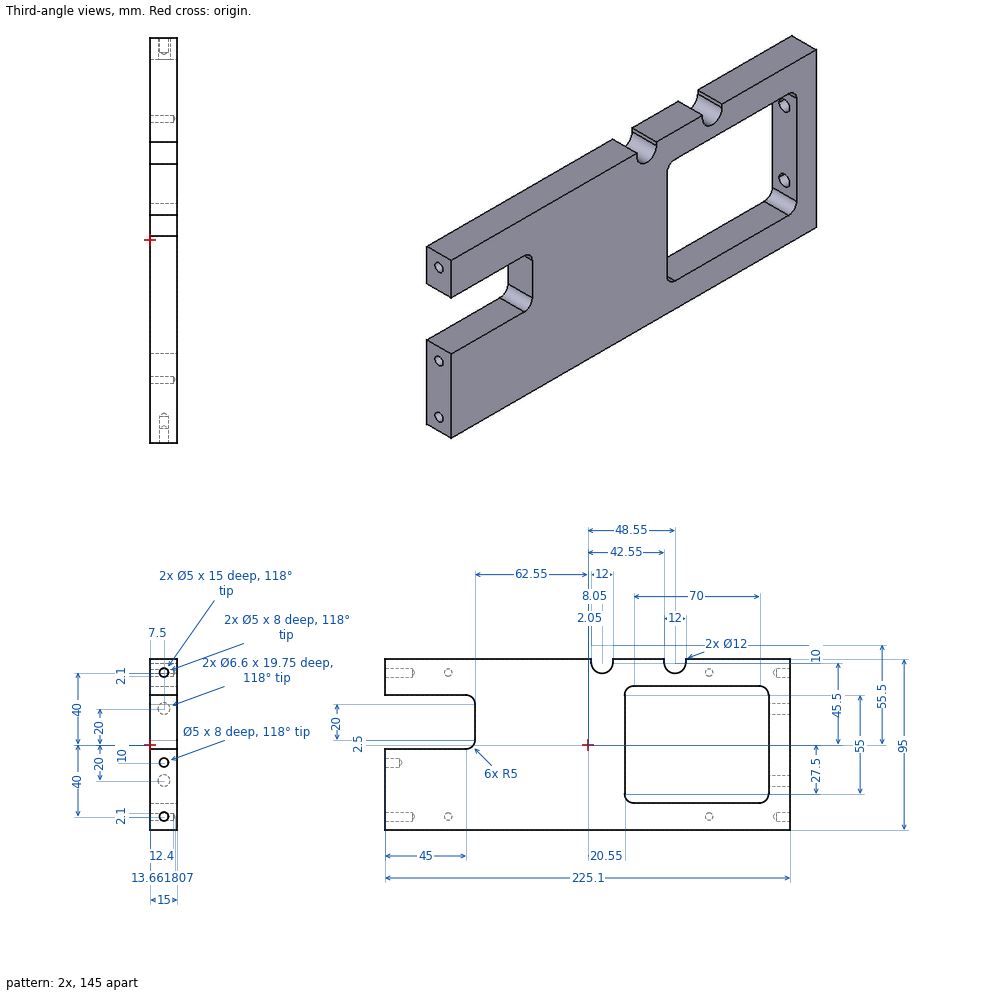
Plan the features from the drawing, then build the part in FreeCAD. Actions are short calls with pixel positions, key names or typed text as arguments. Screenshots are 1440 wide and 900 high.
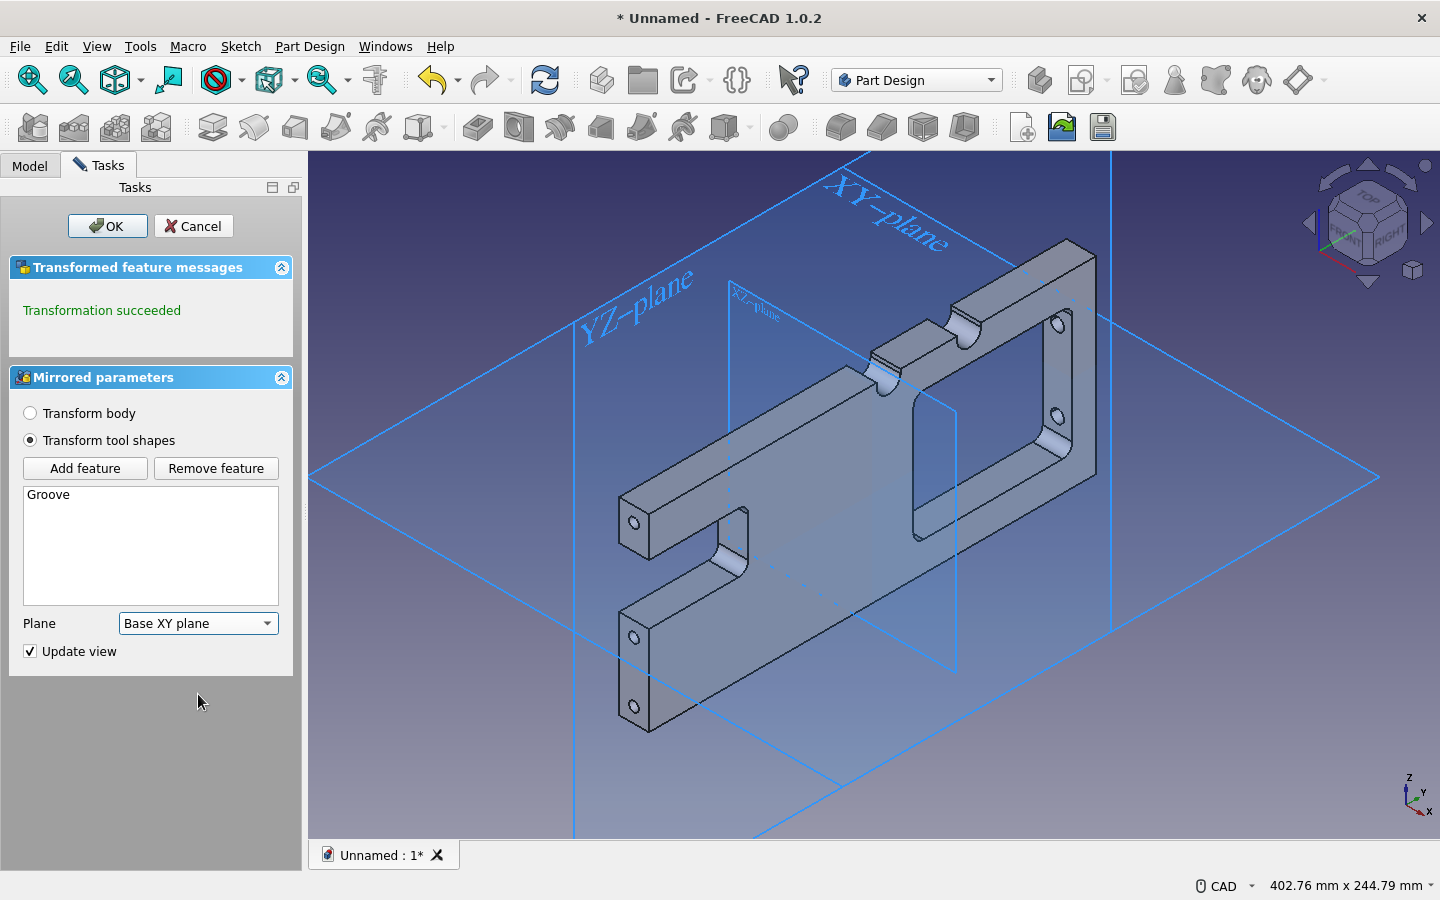
click(108, 226)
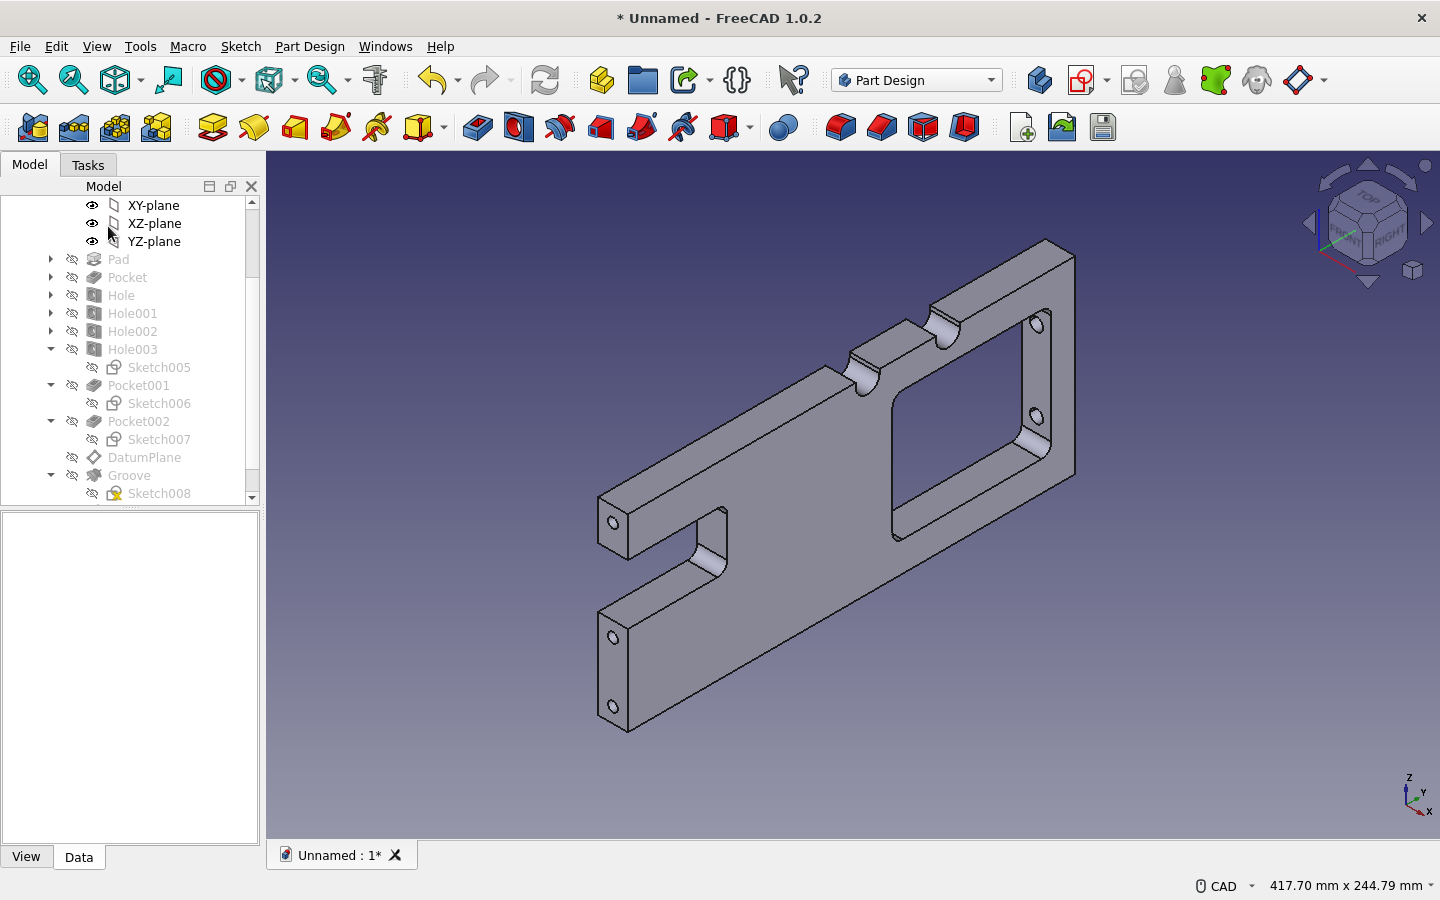
scroll(161, 345, down, 3)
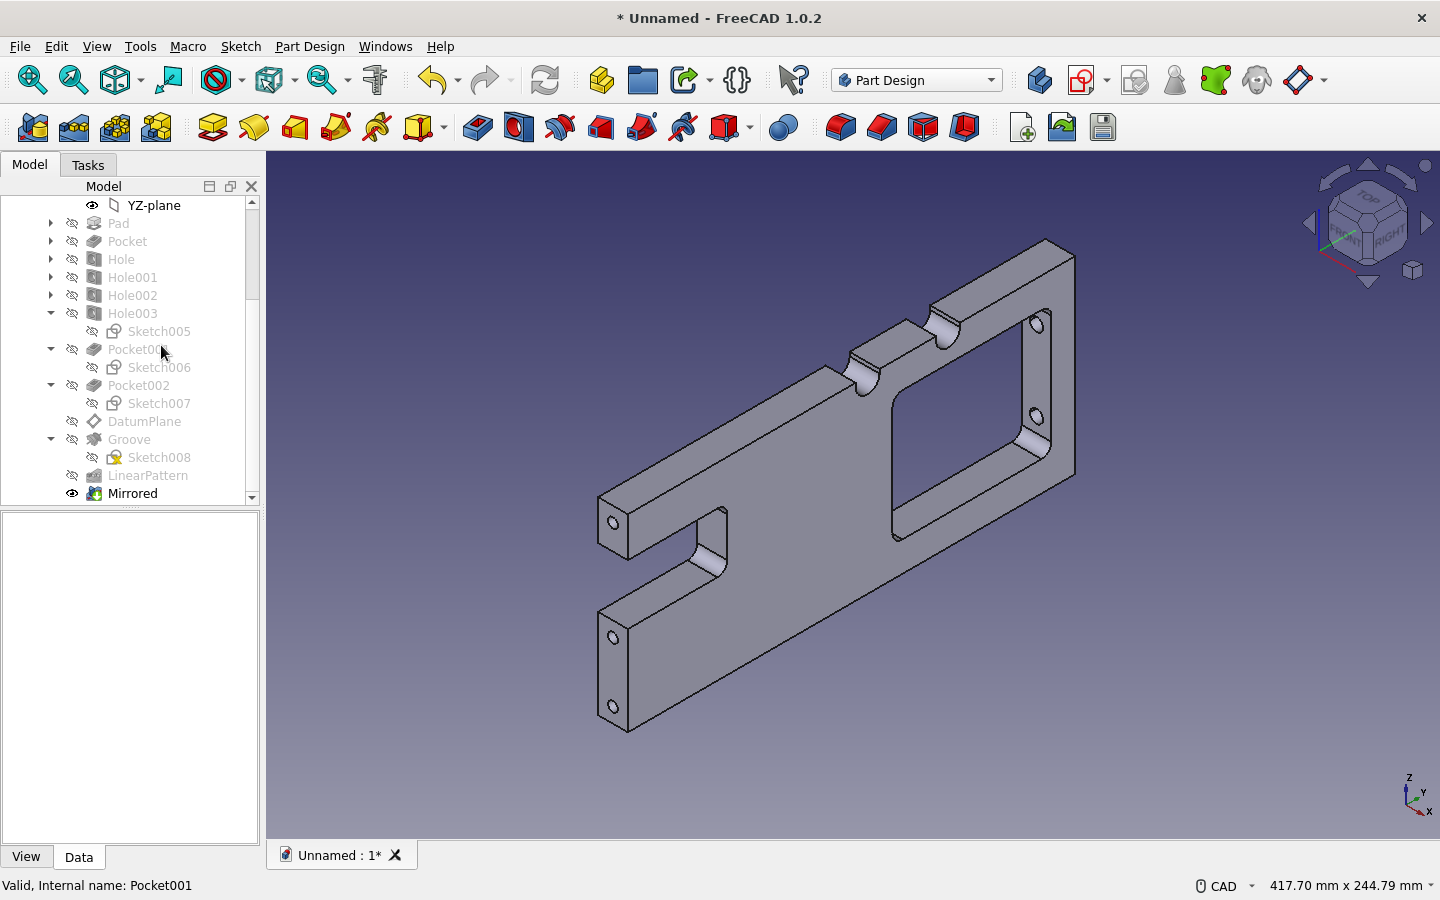
scroll(161, 345, up, 15)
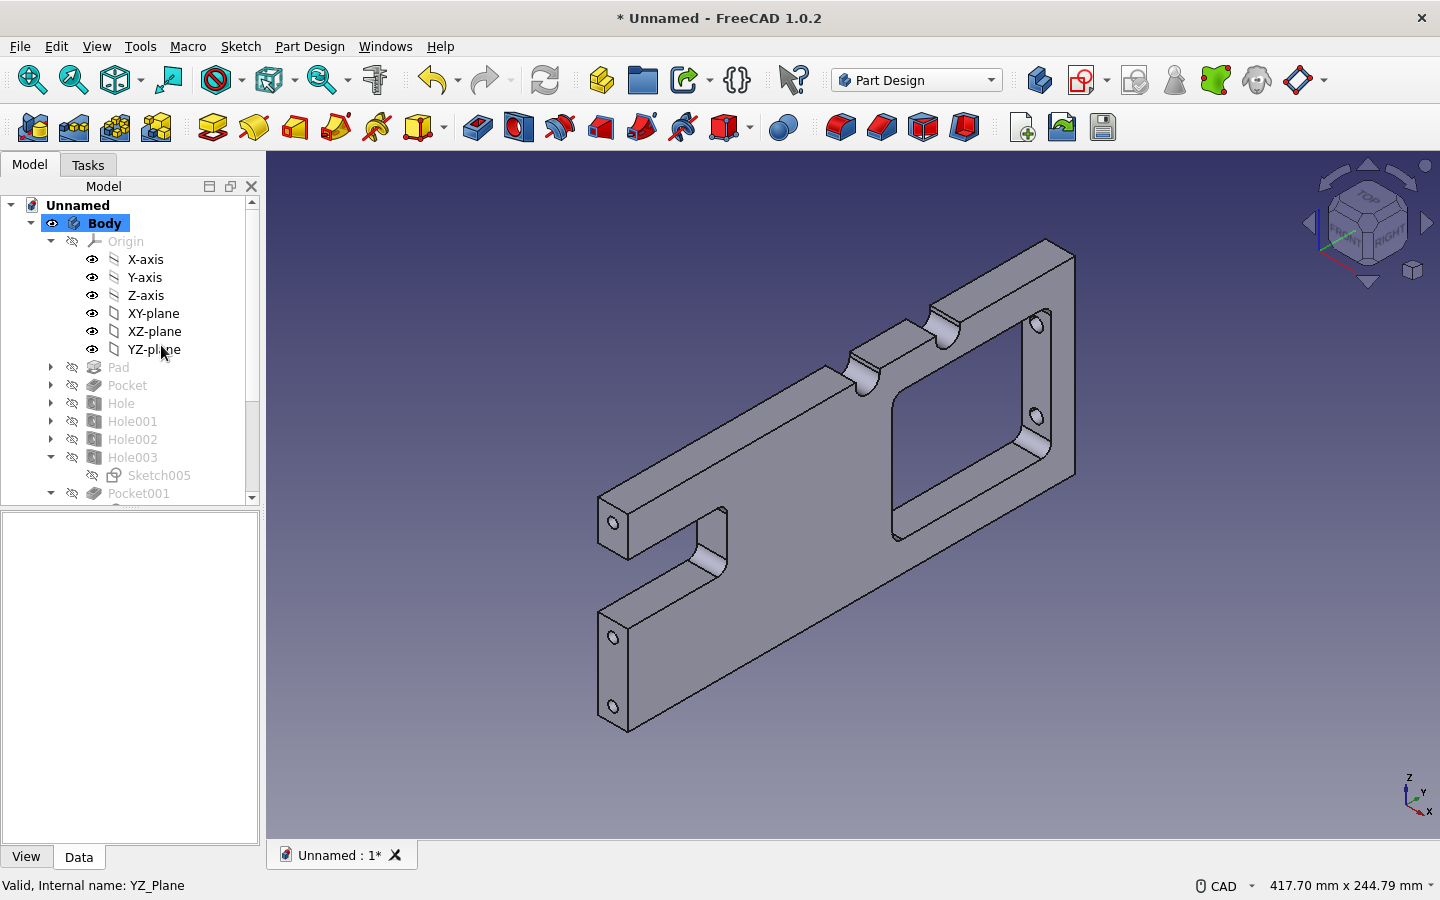
click(137, 331)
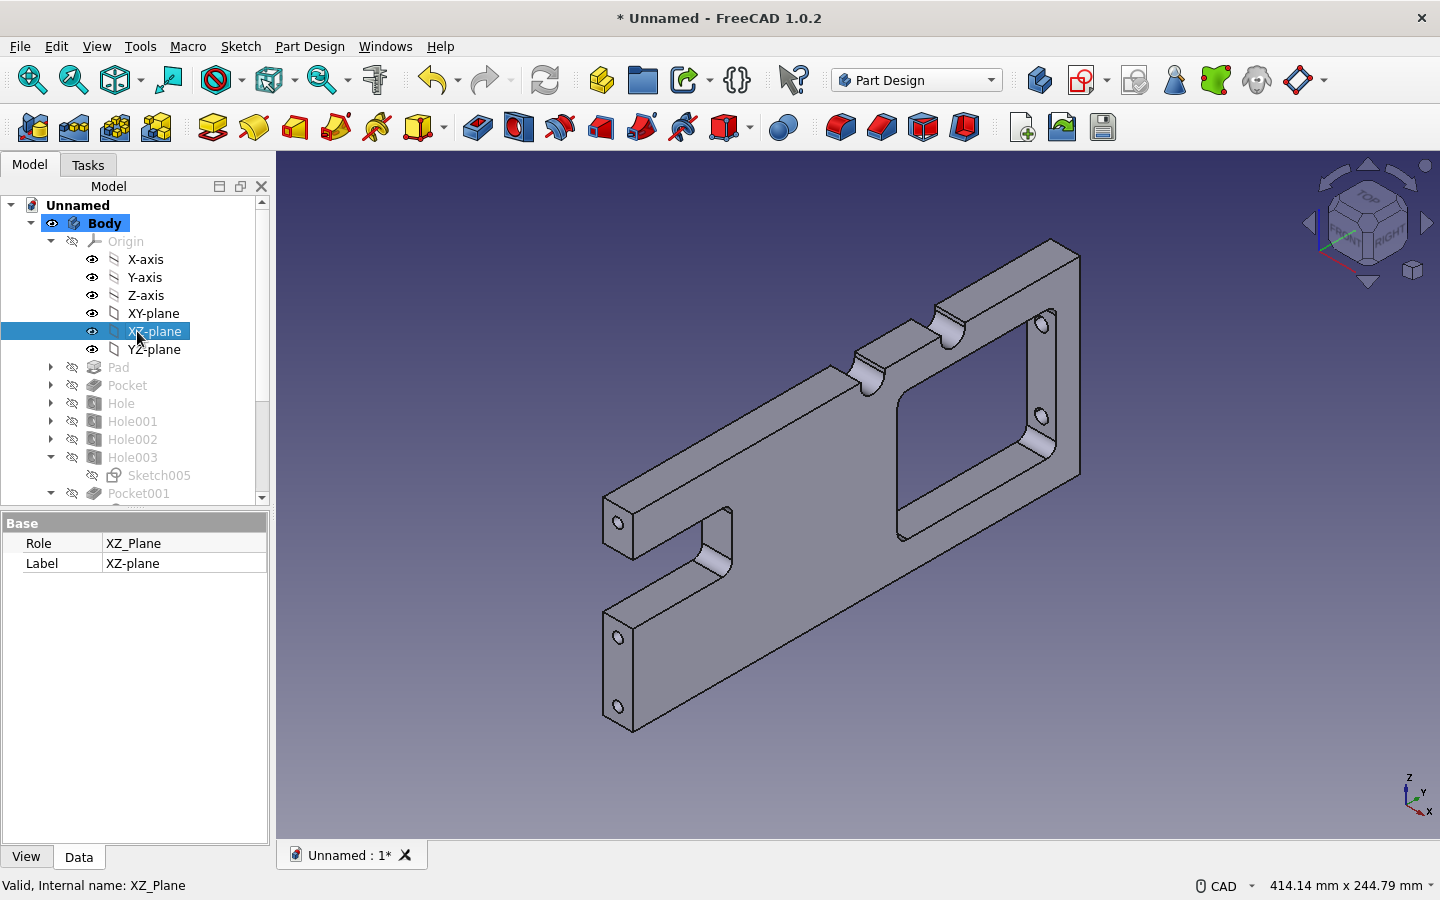
click(1298, 80)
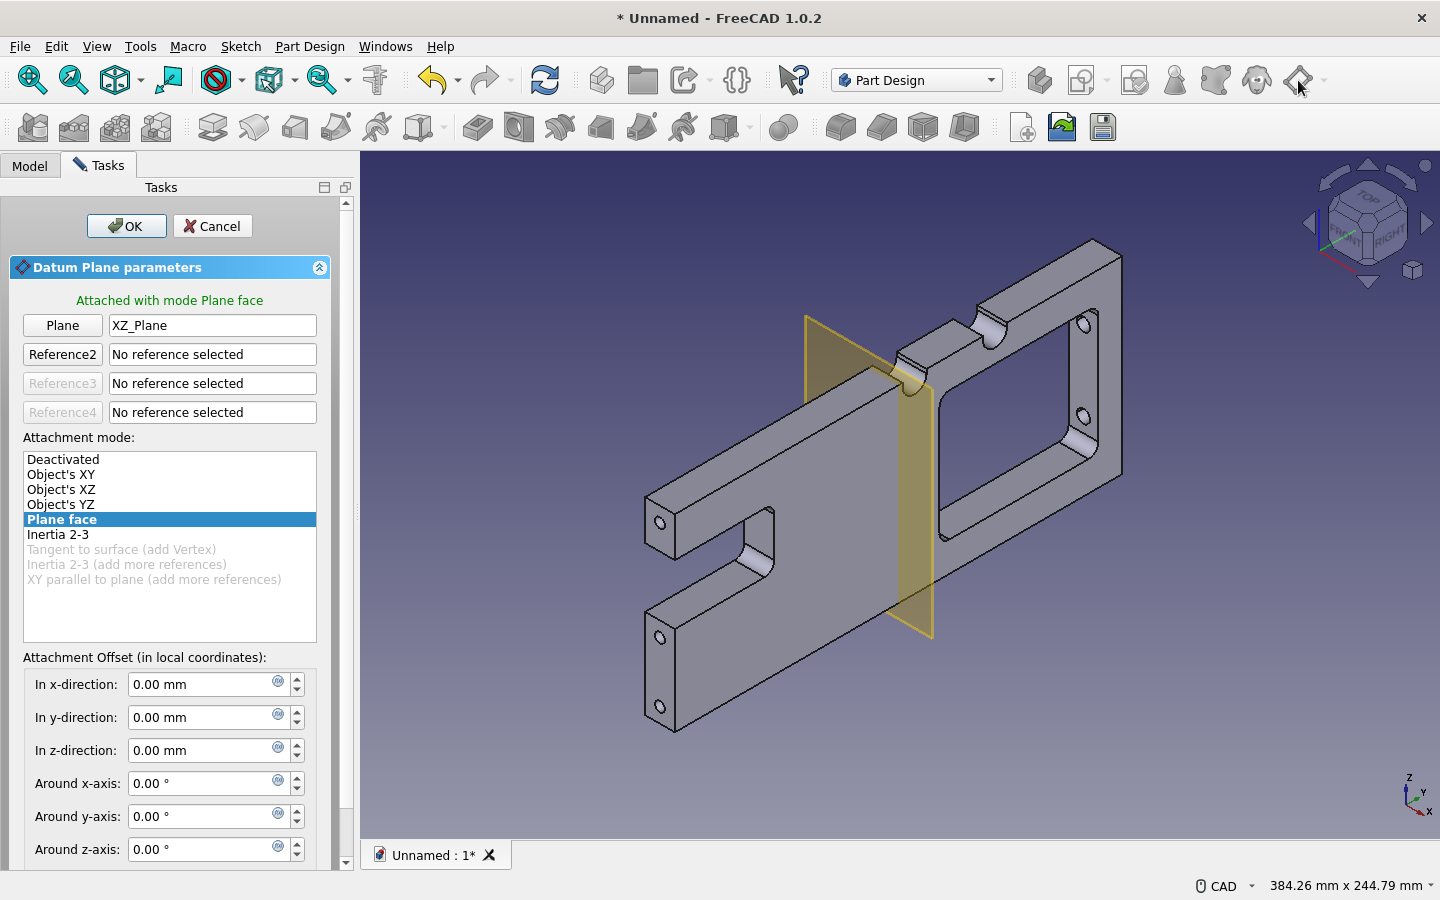
triple_click(210, 750)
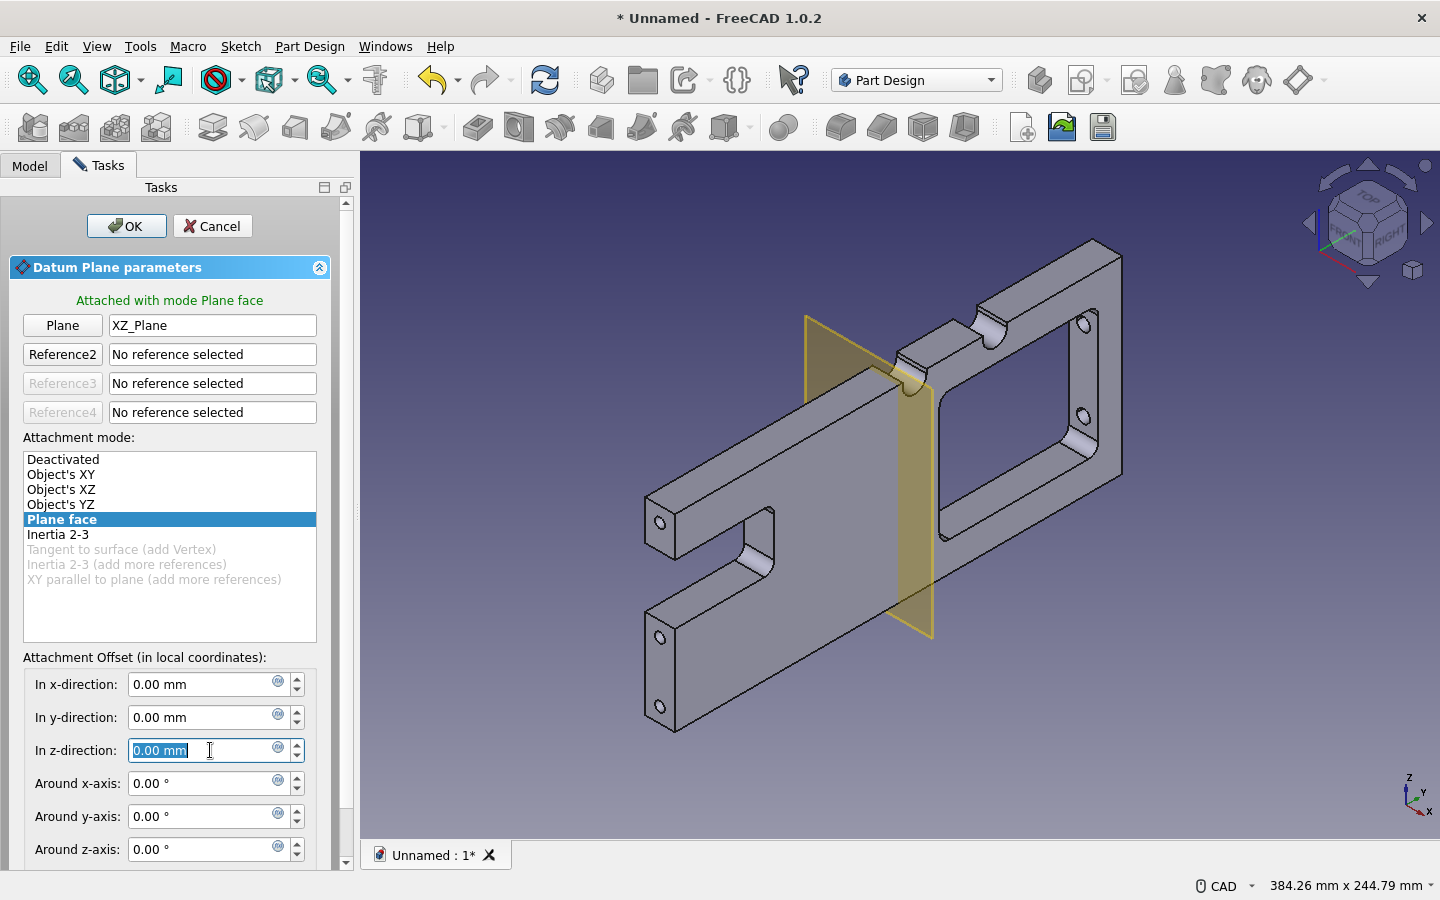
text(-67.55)
key(Tab)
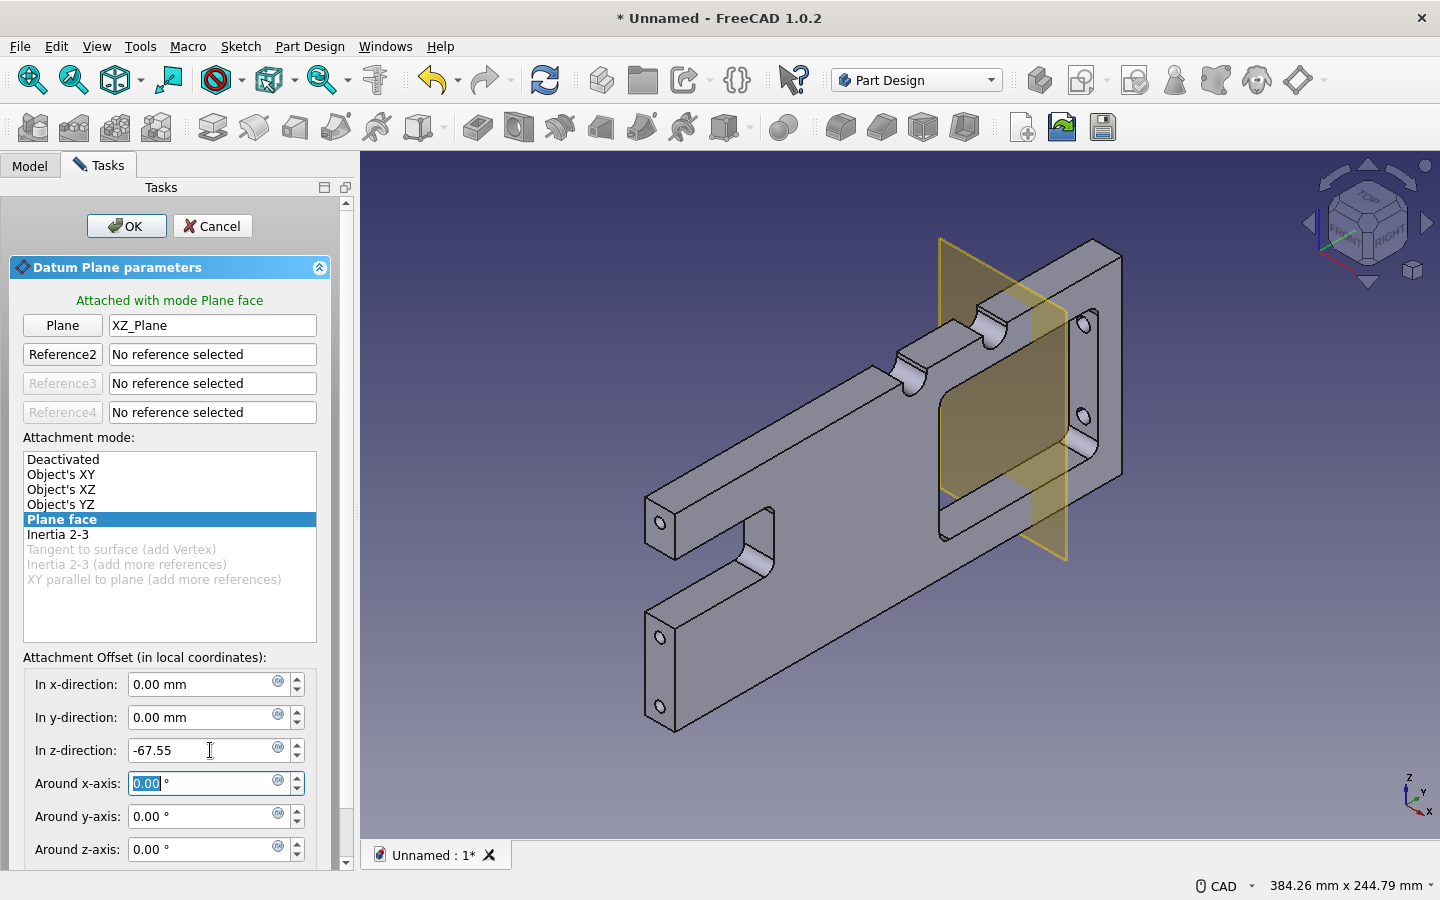
click(127, 226)